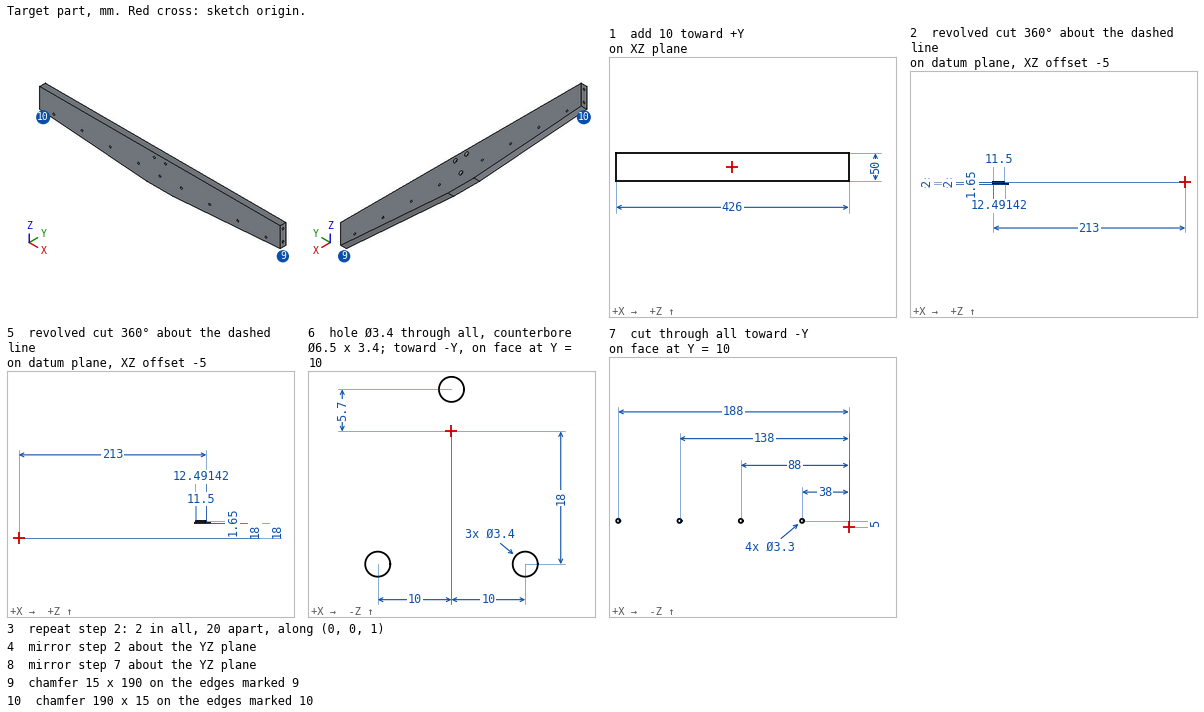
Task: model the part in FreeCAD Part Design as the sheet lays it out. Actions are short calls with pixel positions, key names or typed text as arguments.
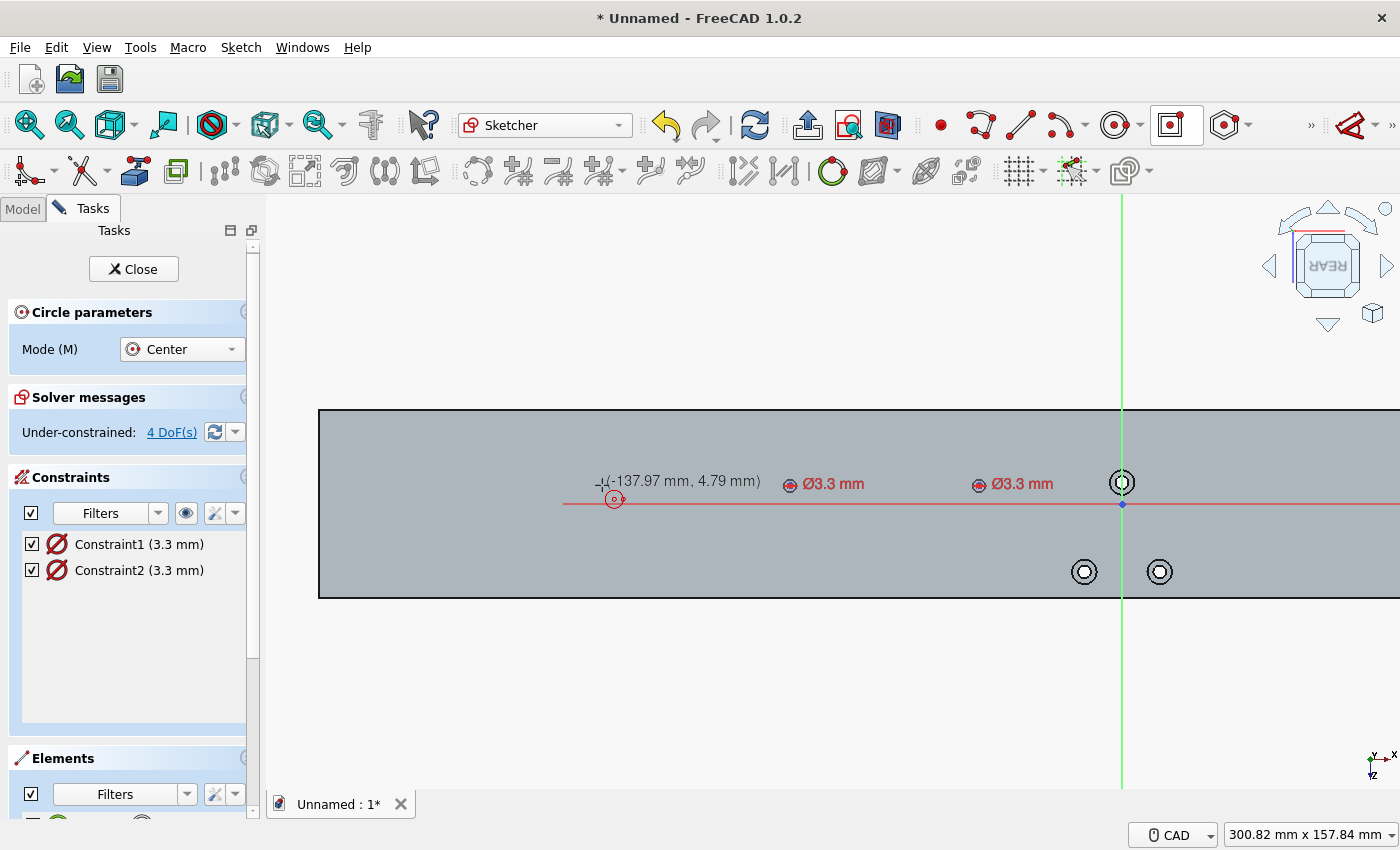
click(602, 485)
move(606, 481)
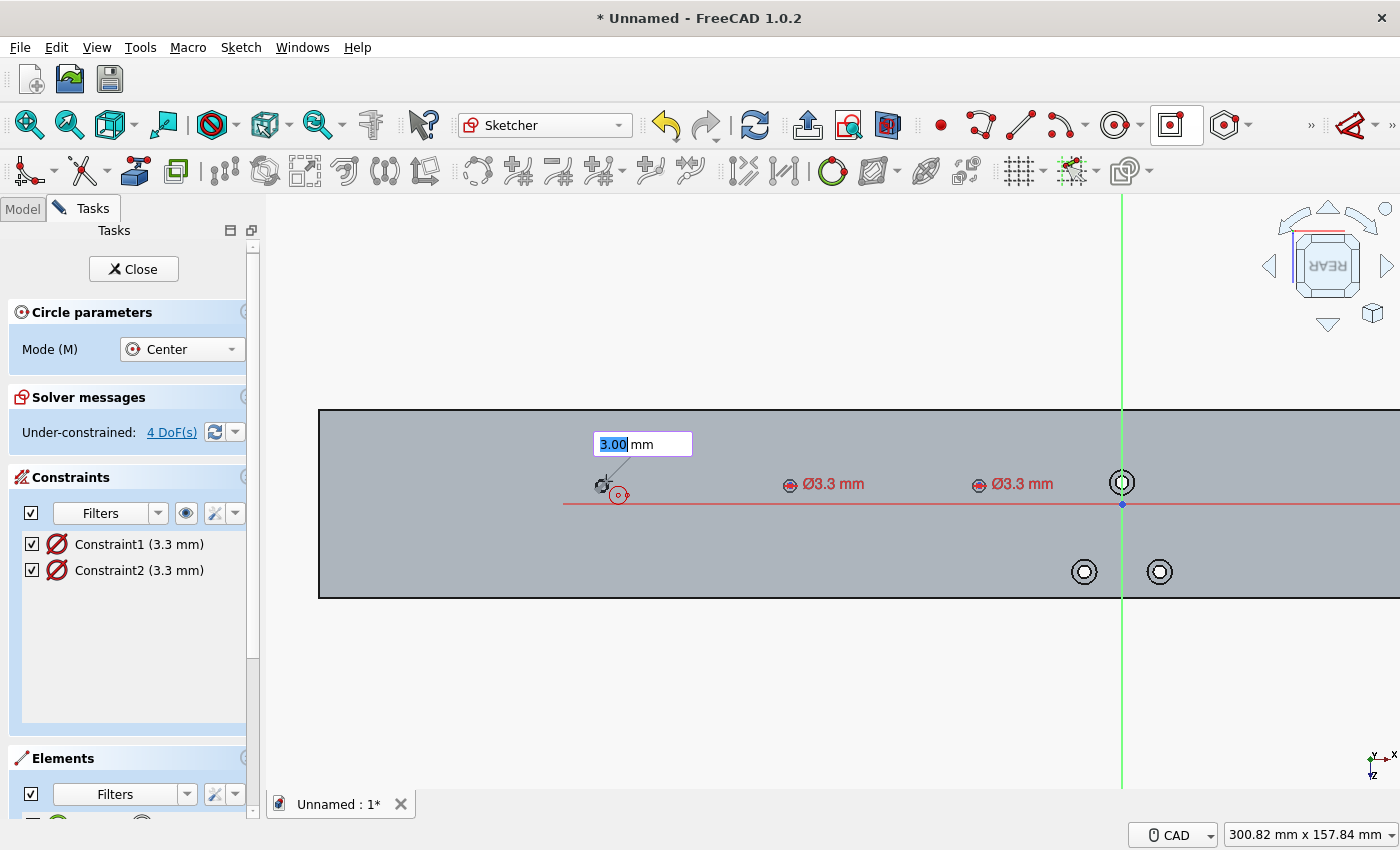
text(3.3)
key(Return)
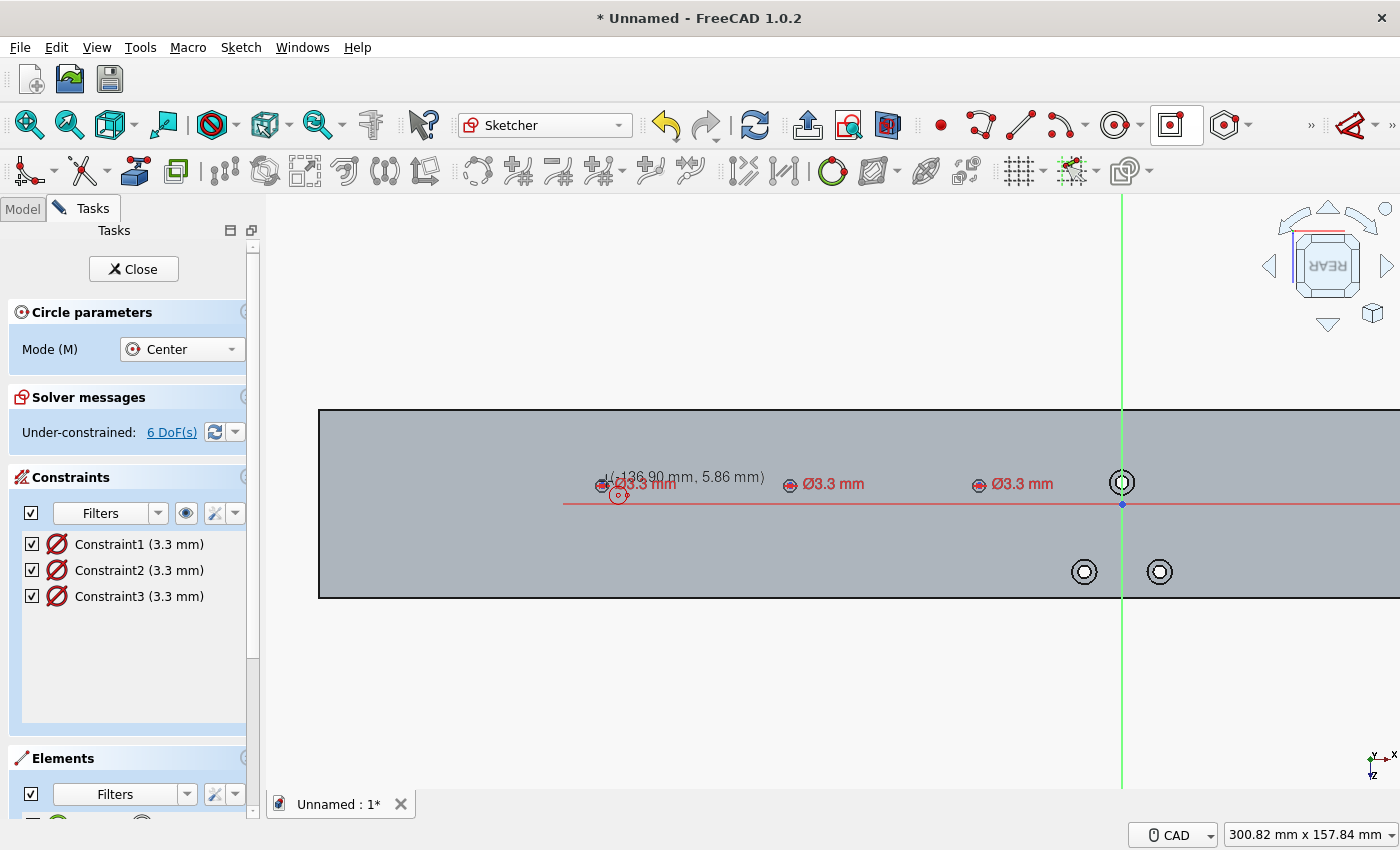
scroll(413, 485, up, 7)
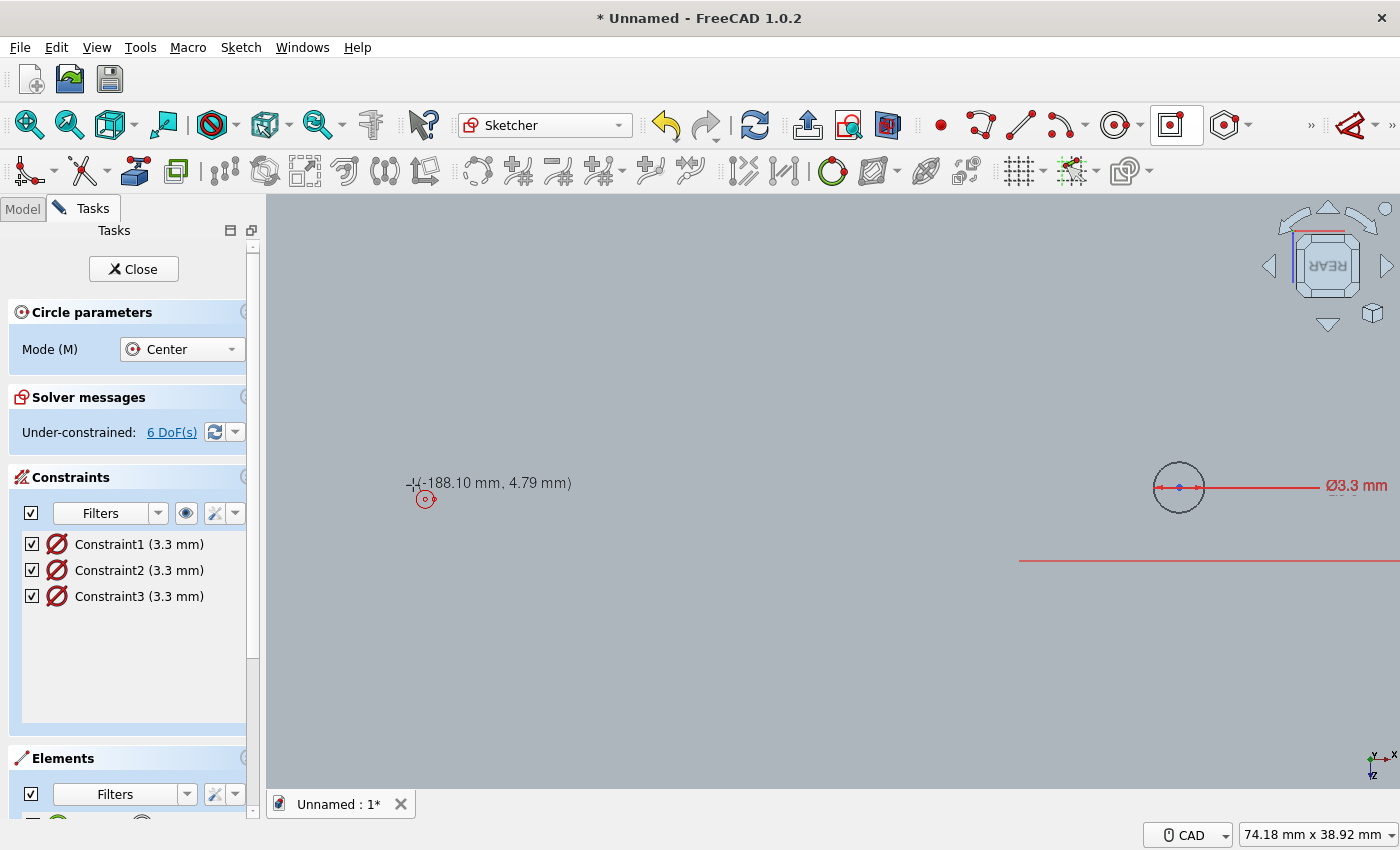
scroll(413, 485, down, 7)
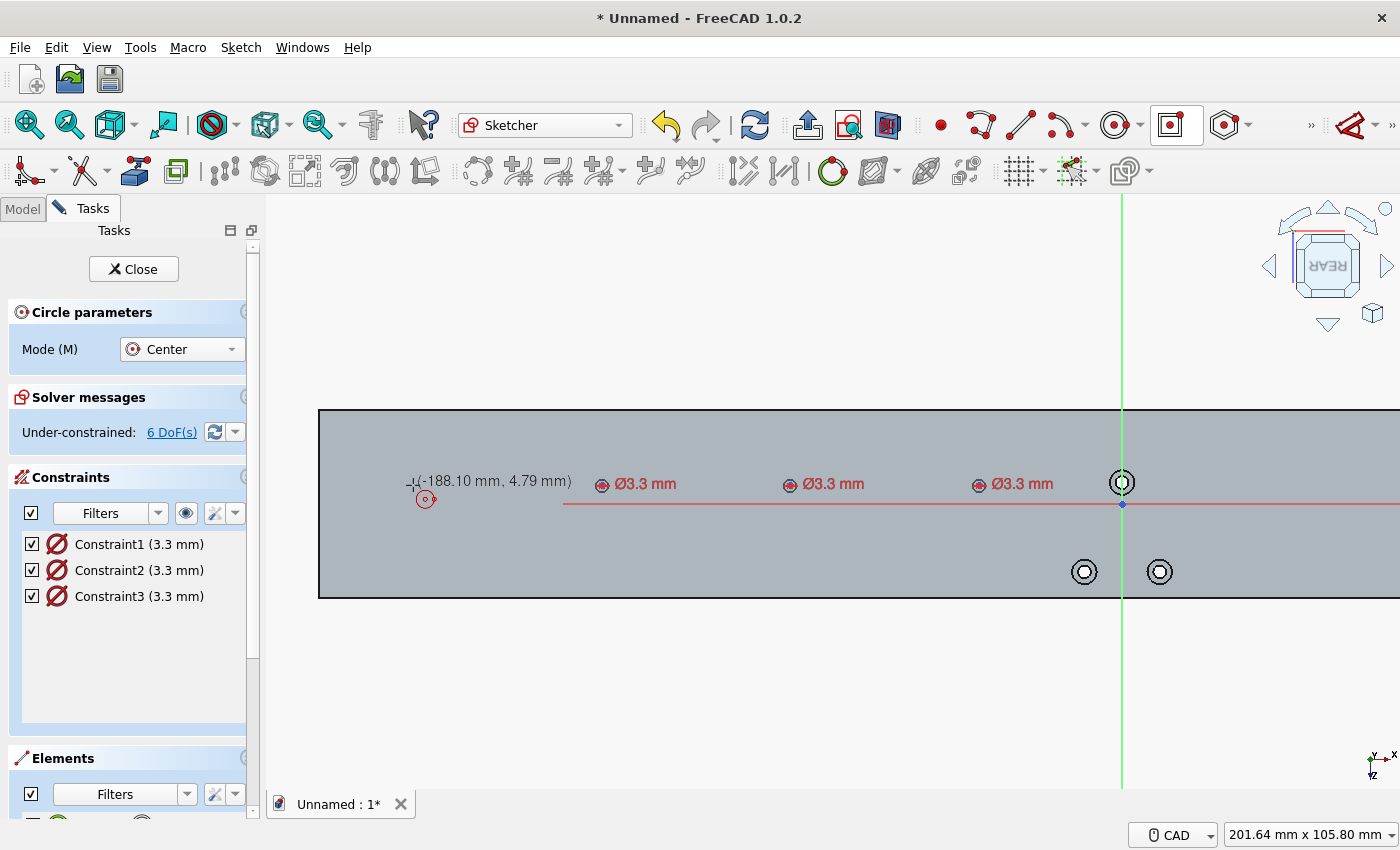
click(413, 485)
move(418, 481)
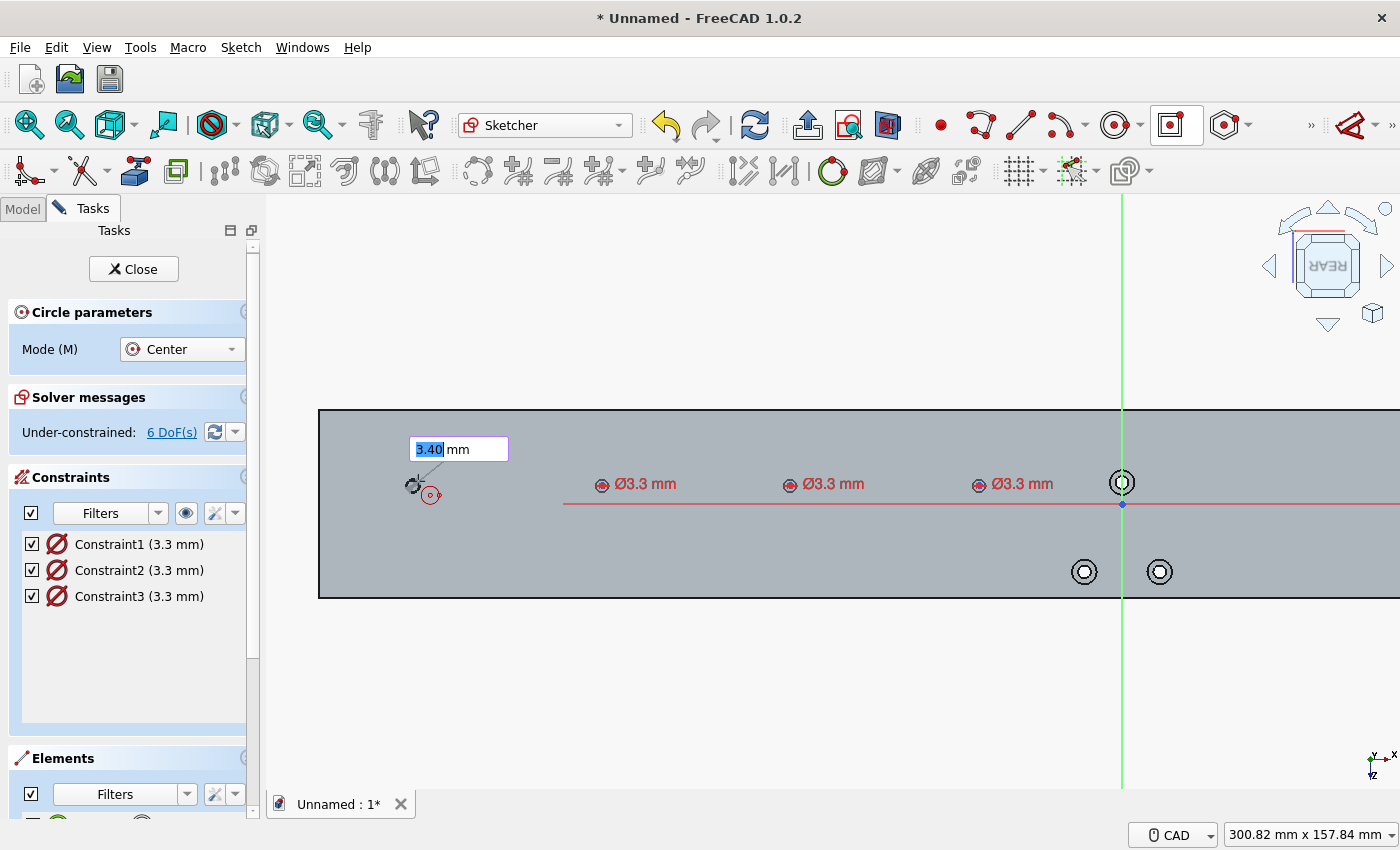
text(3.3)
key(Return)
key(Escape)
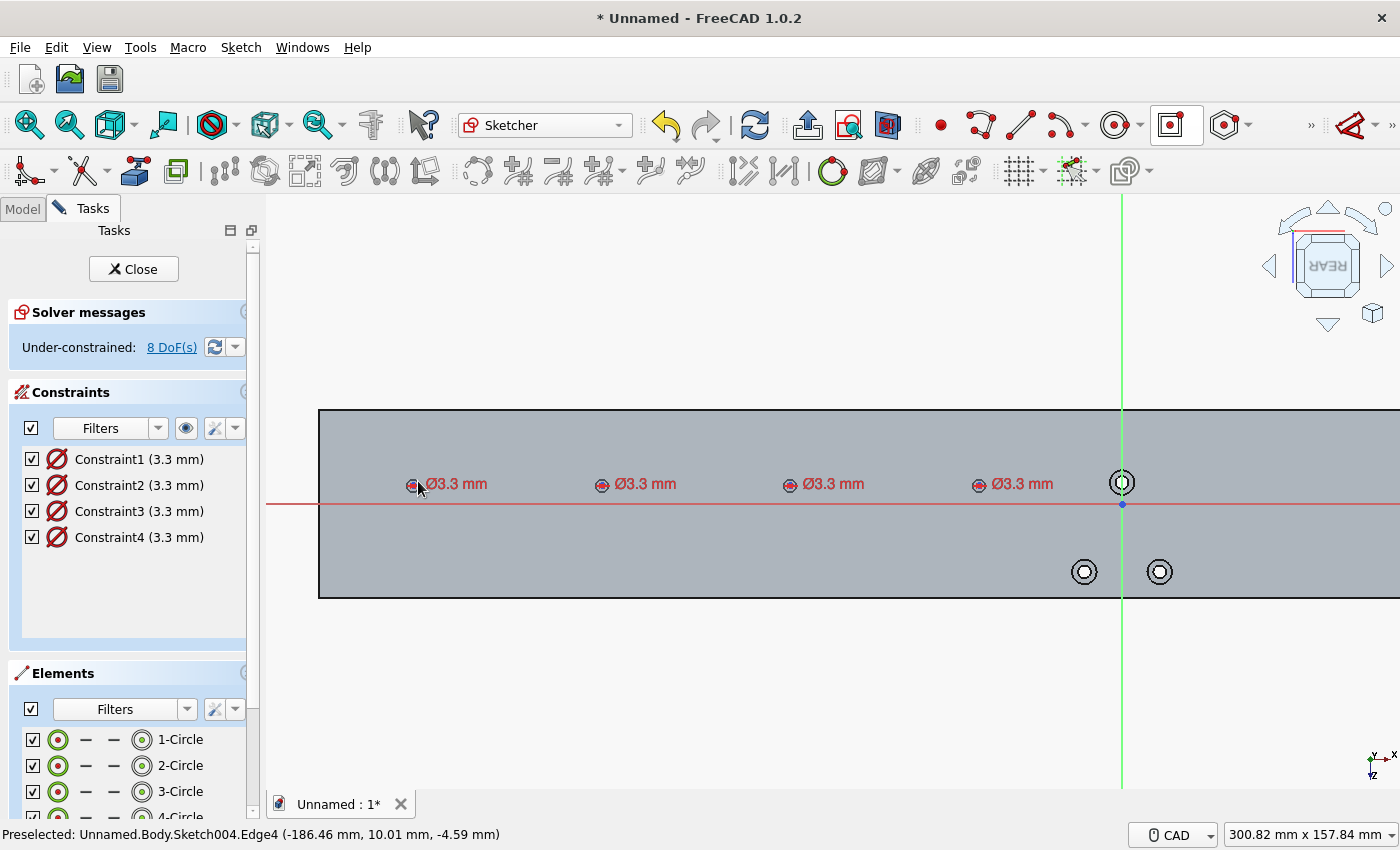
click(979, 486)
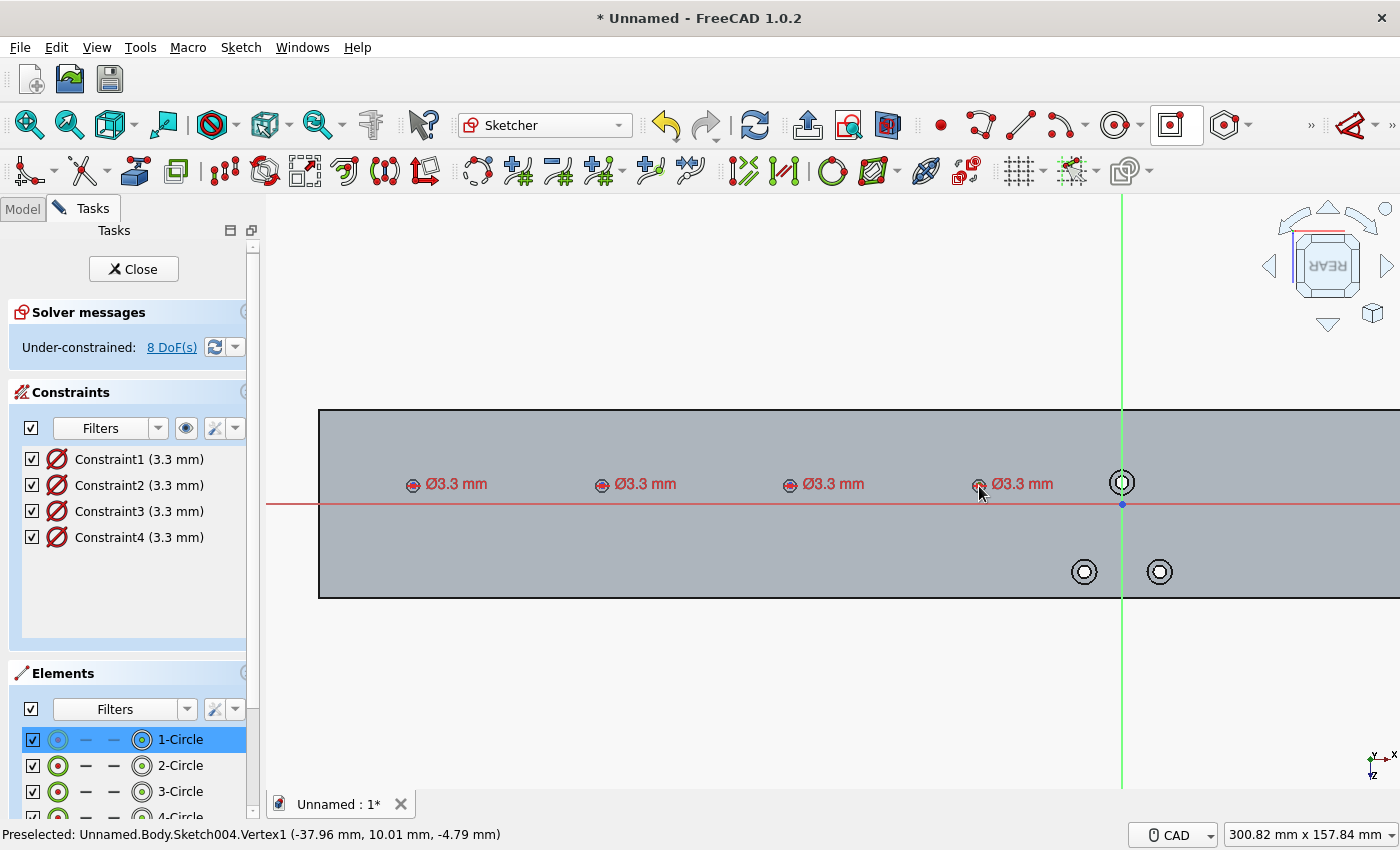
click(790, 486)